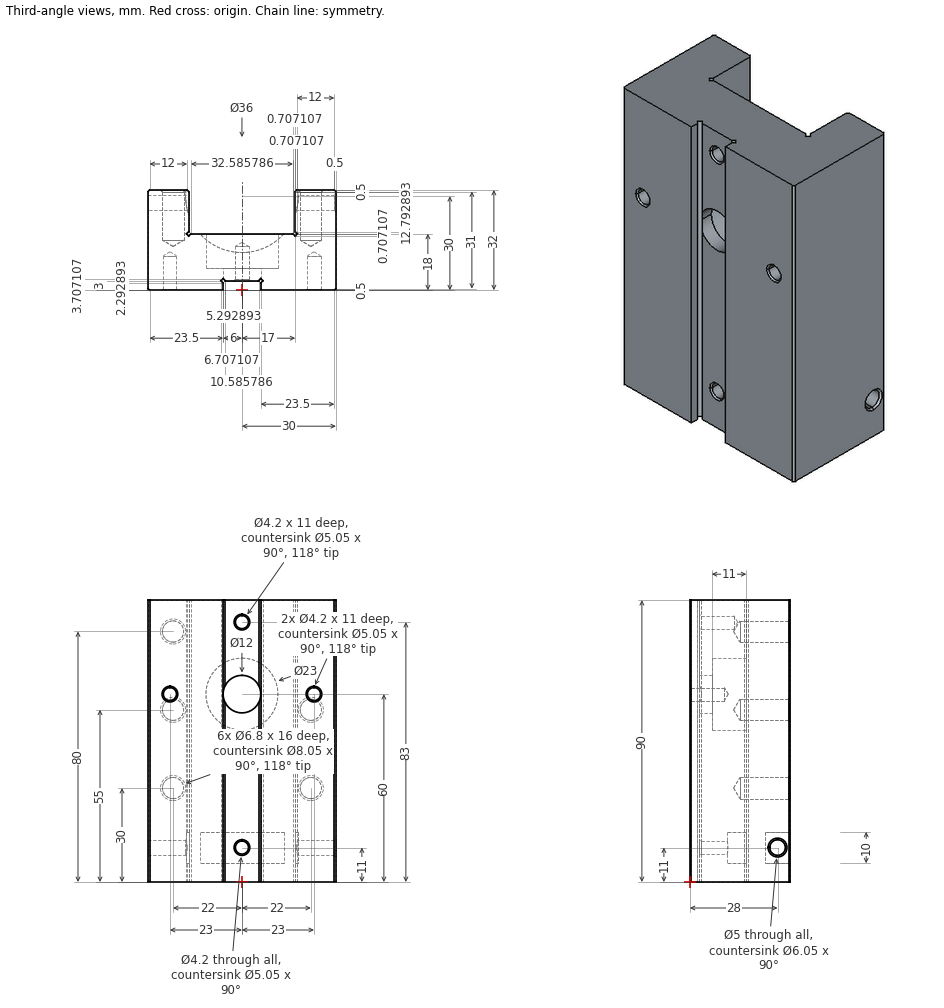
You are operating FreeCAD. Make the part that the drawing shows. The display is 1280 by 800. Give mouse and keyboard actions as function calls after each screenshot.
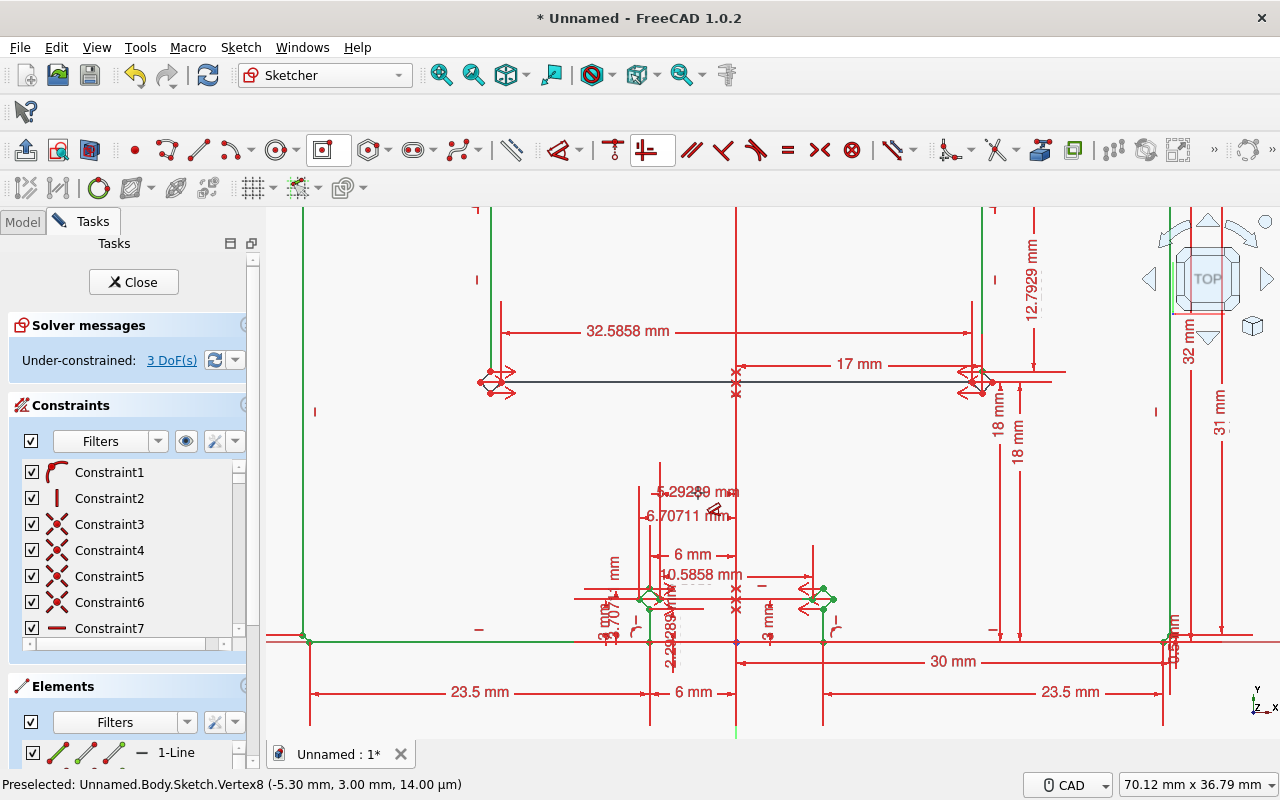
scroll(987, 377, up, 7)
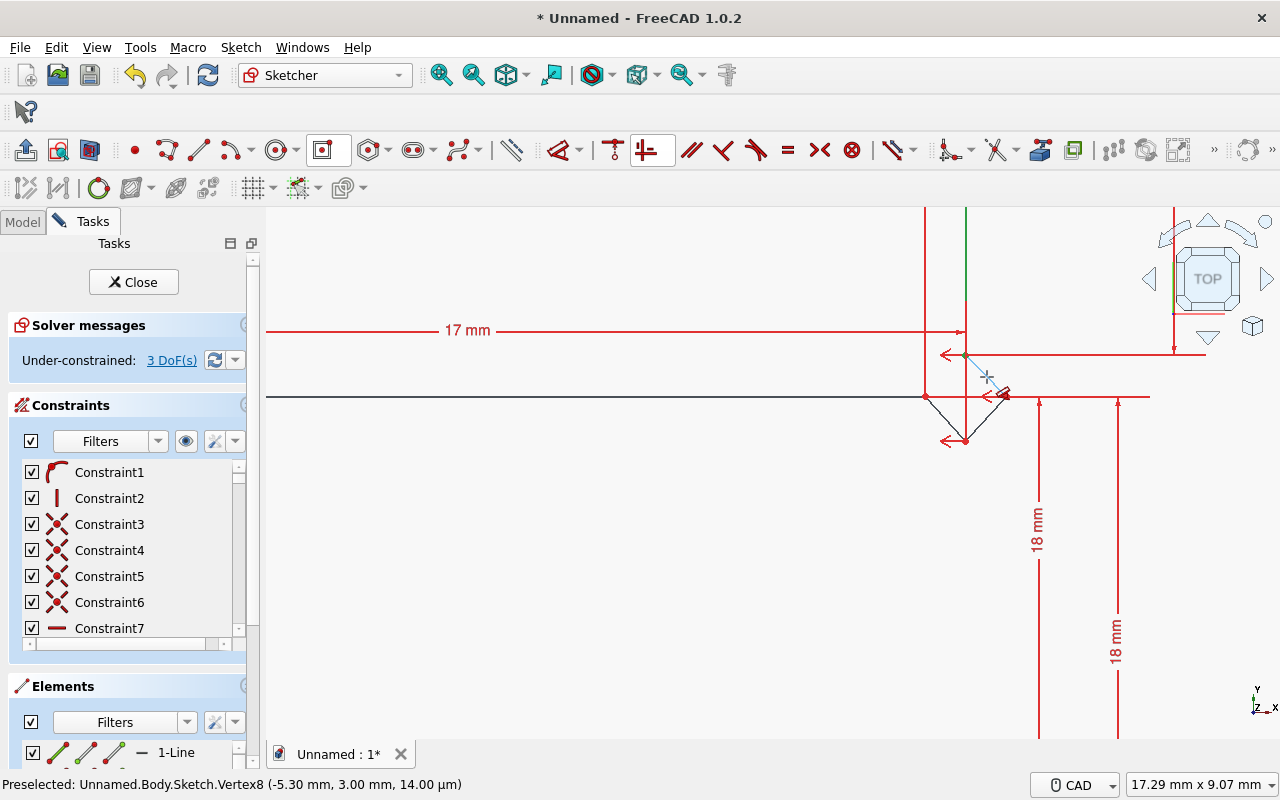
click(986, 376)
click(986, 321)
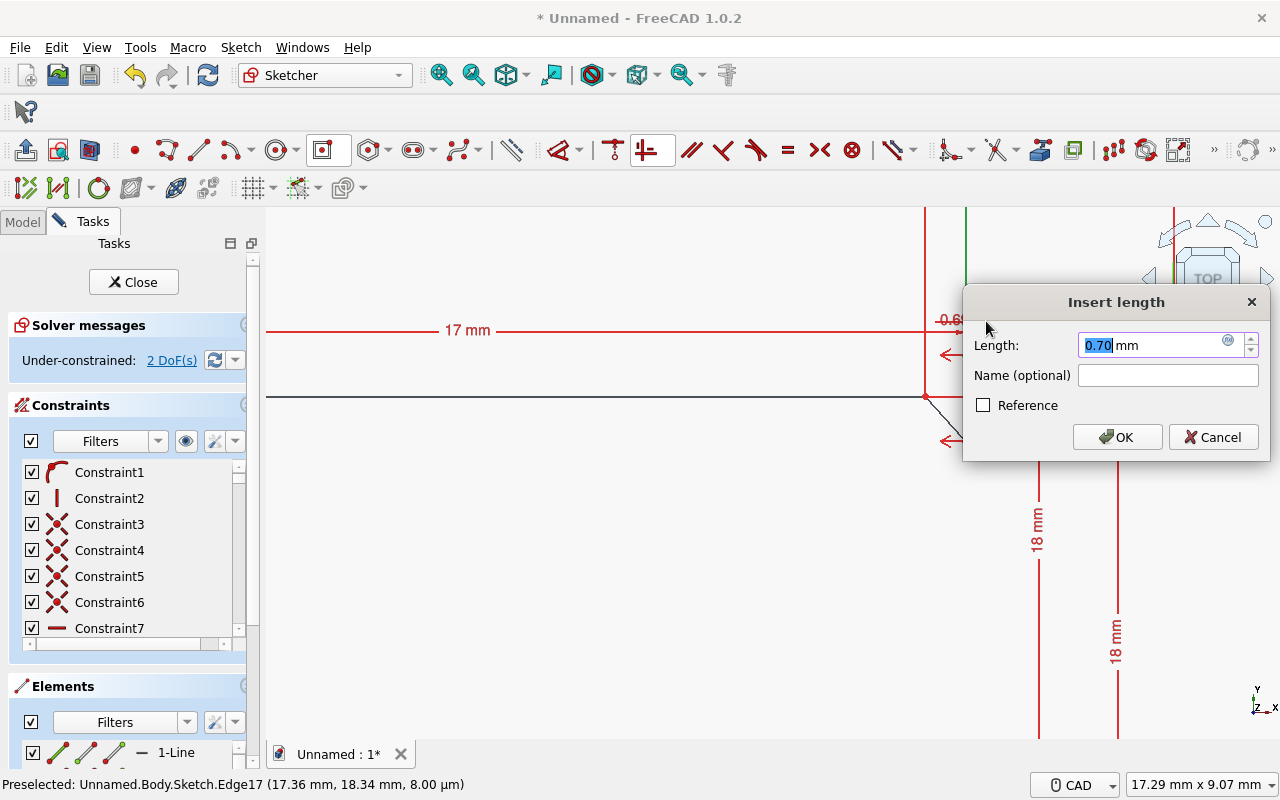
text(0.707107)
key(Return)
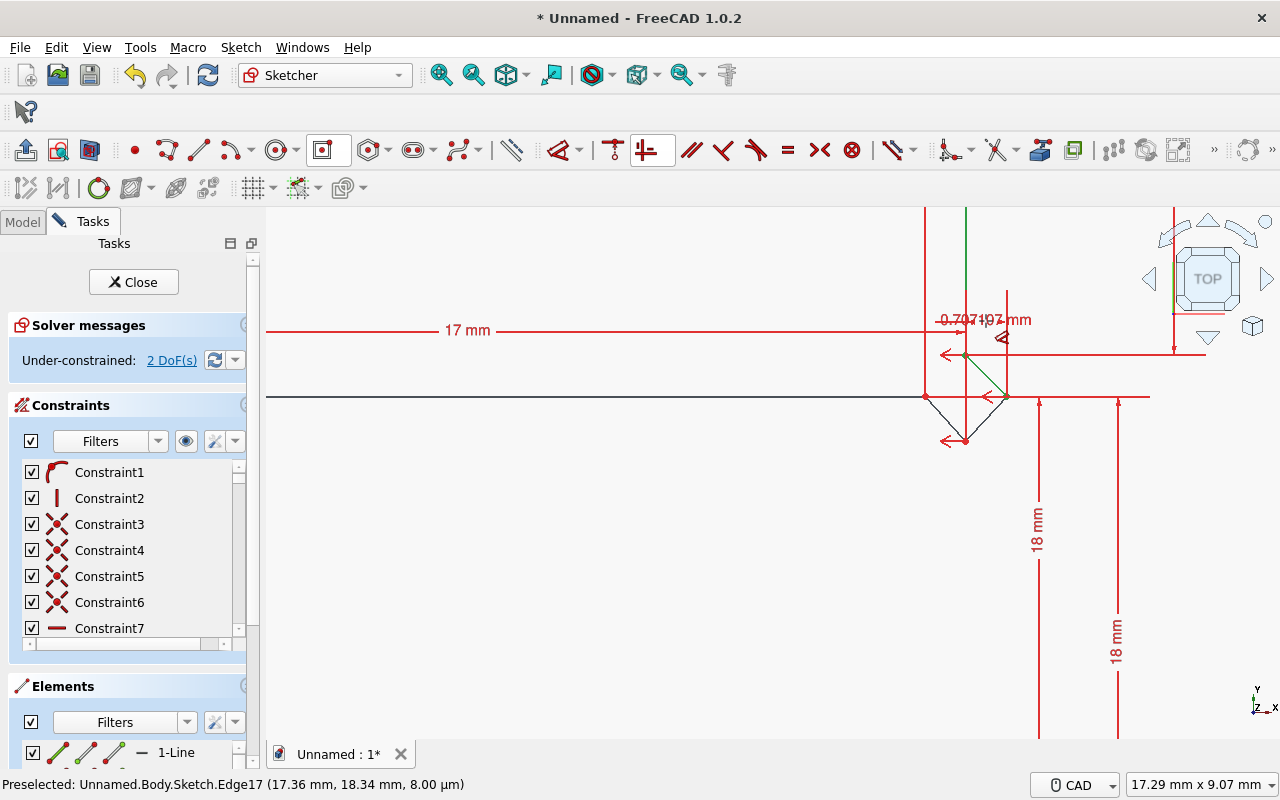
click(995, 410)
click(1041, 419)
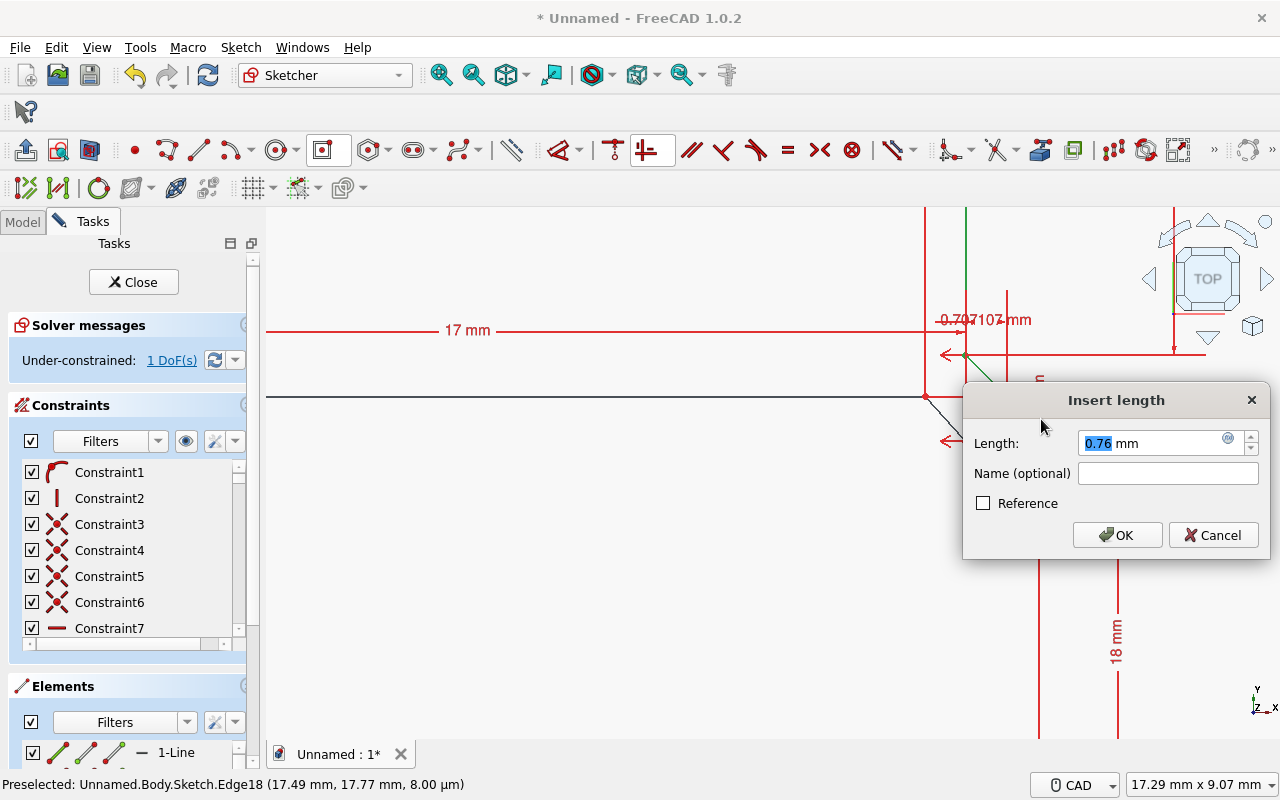
text(0.707107)
key(Return)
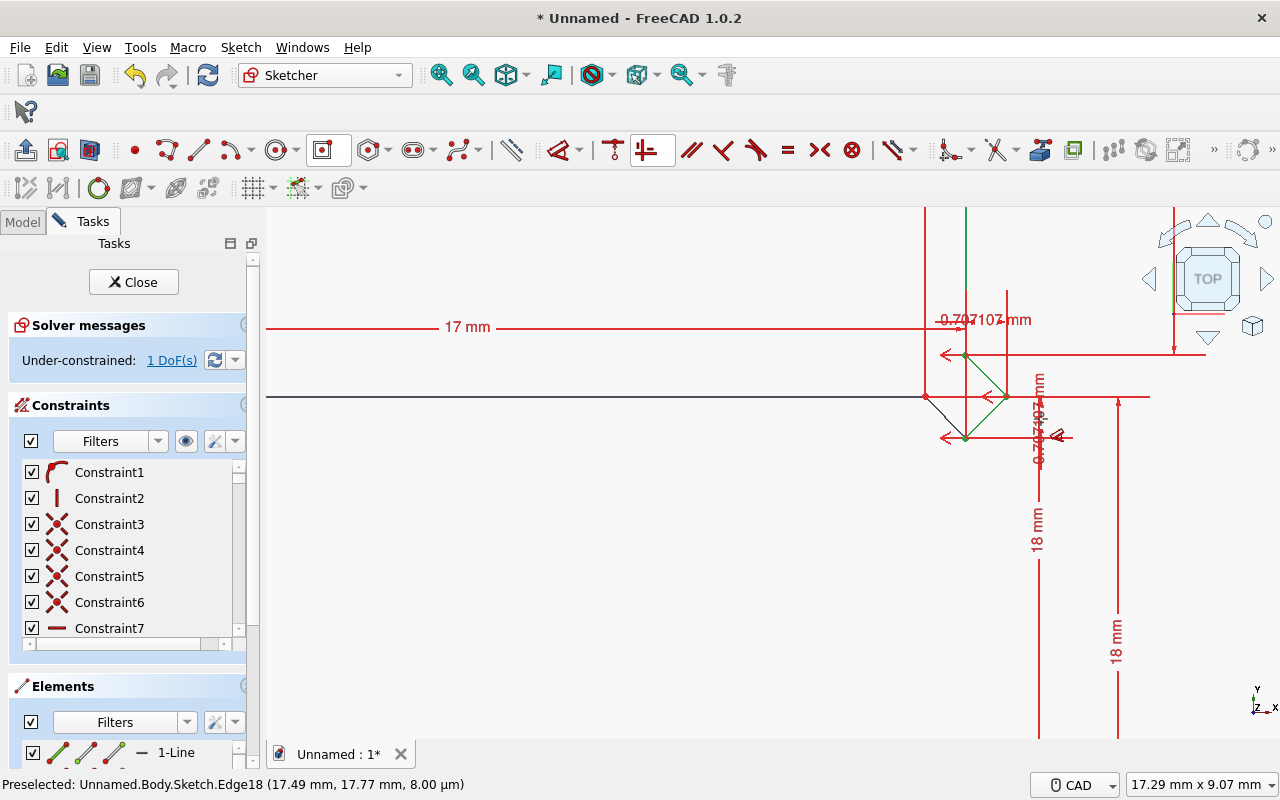
click(953, 426)
click(945, 363)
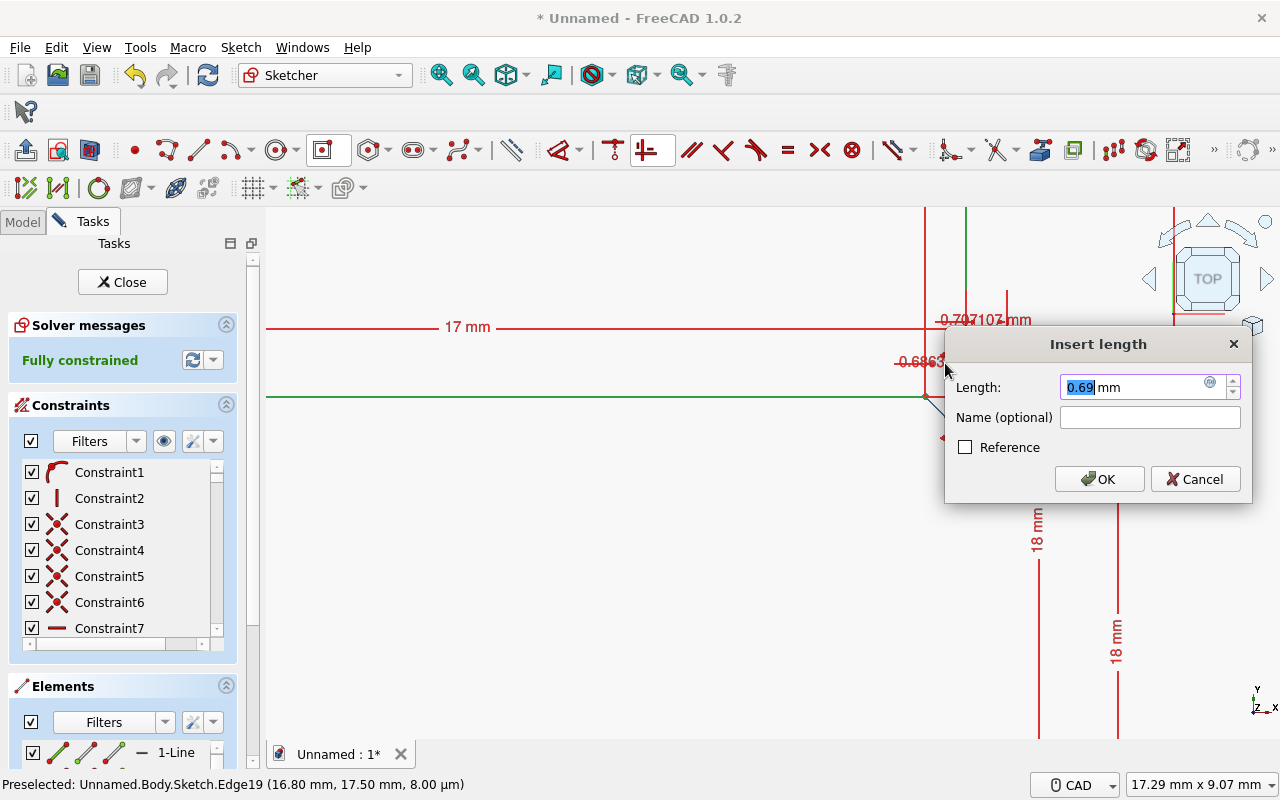
text(0.707107)
key(Return)
key(Escape)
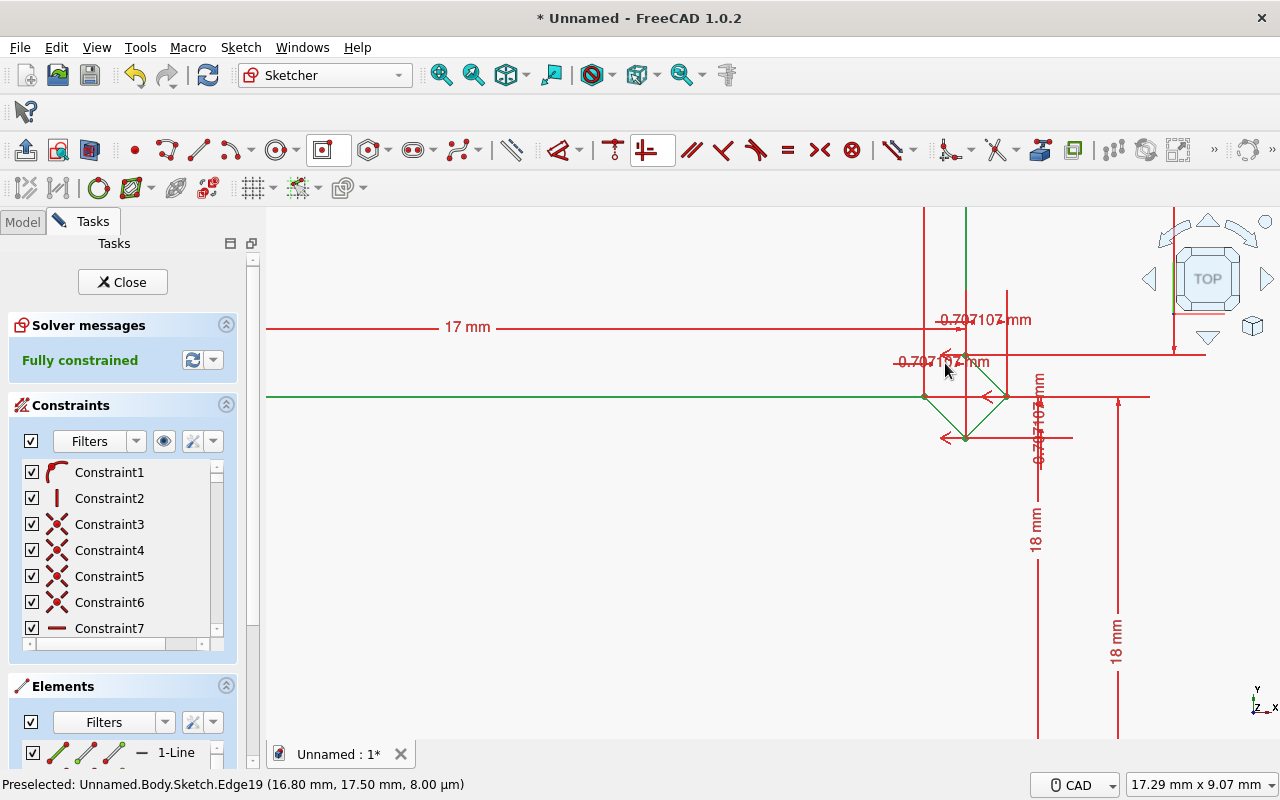
click(123, 282)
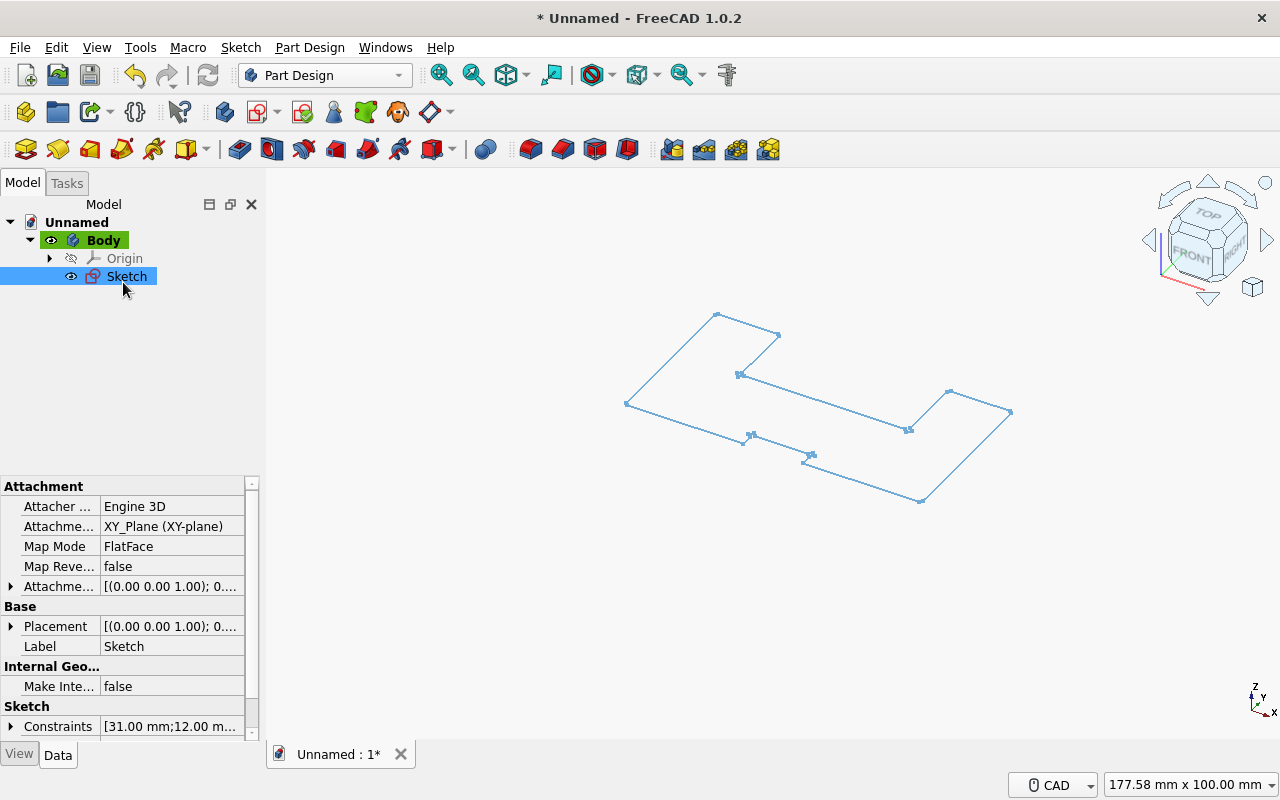
click(26, 150)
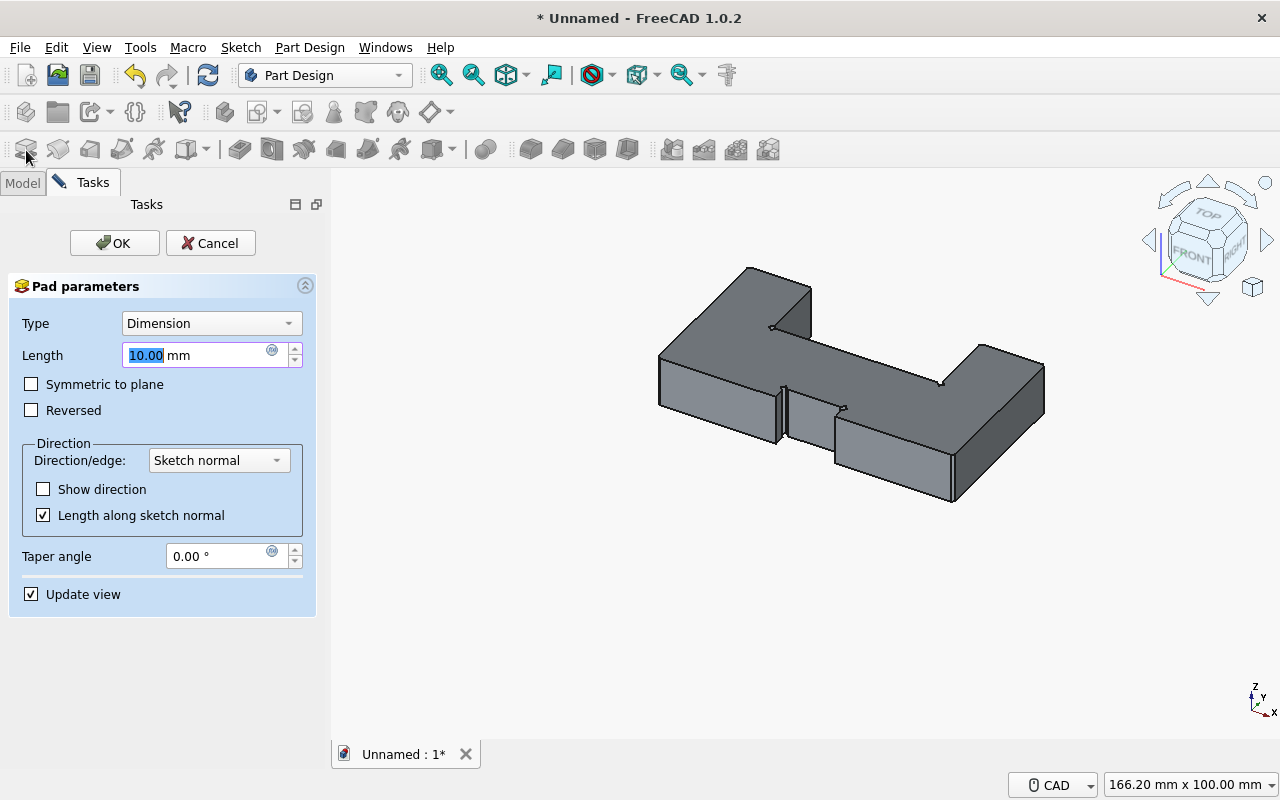
text(90)
key(Tab)